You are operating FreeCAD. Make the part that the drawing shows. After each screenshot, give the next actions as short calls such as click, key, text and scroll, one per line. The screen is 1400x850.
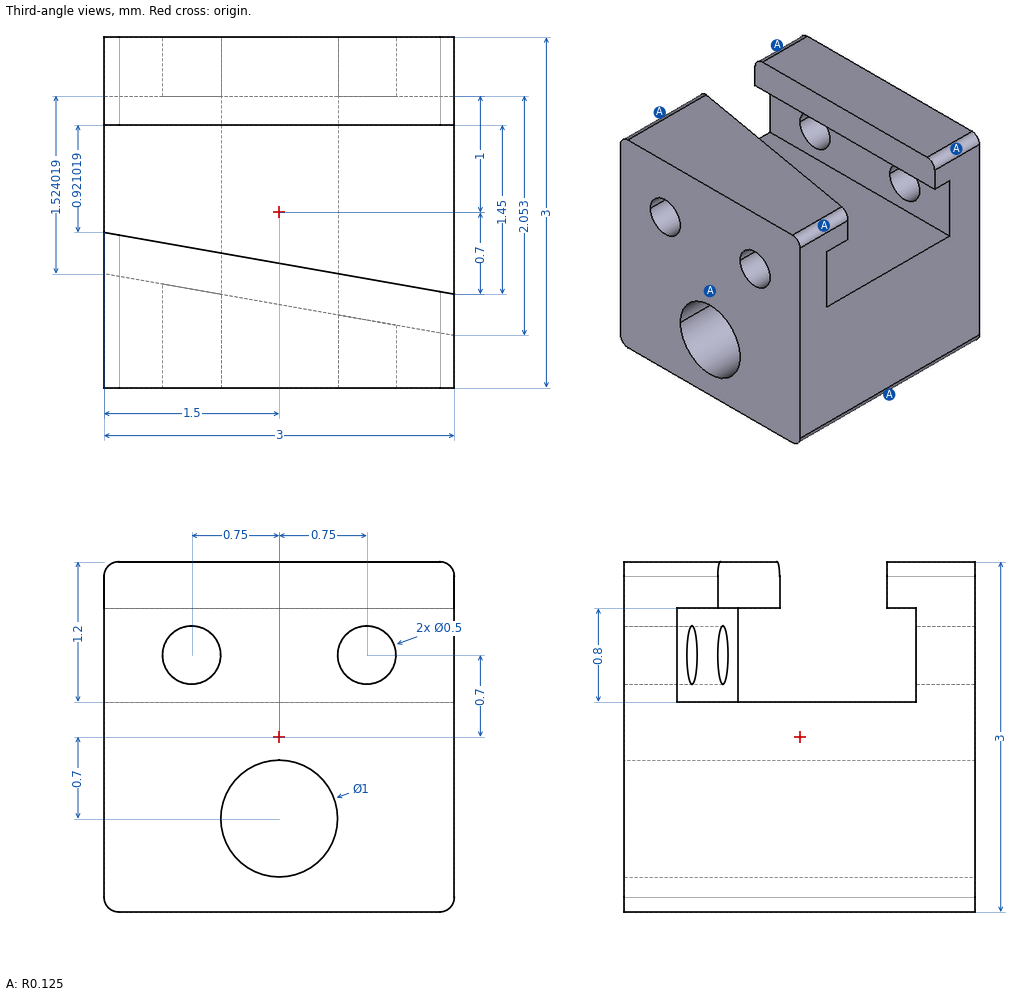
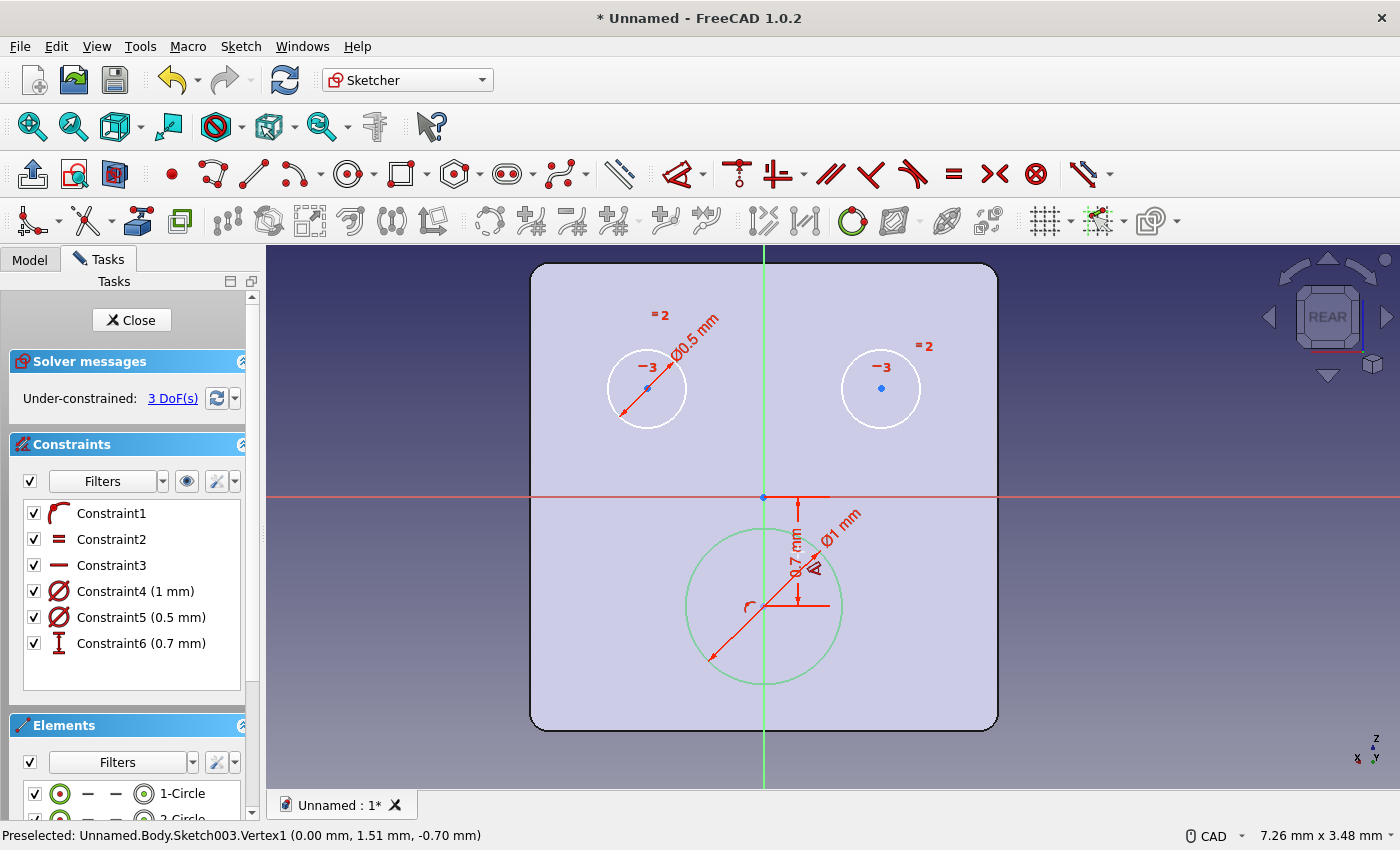
click(647, 389)
click(613, 443)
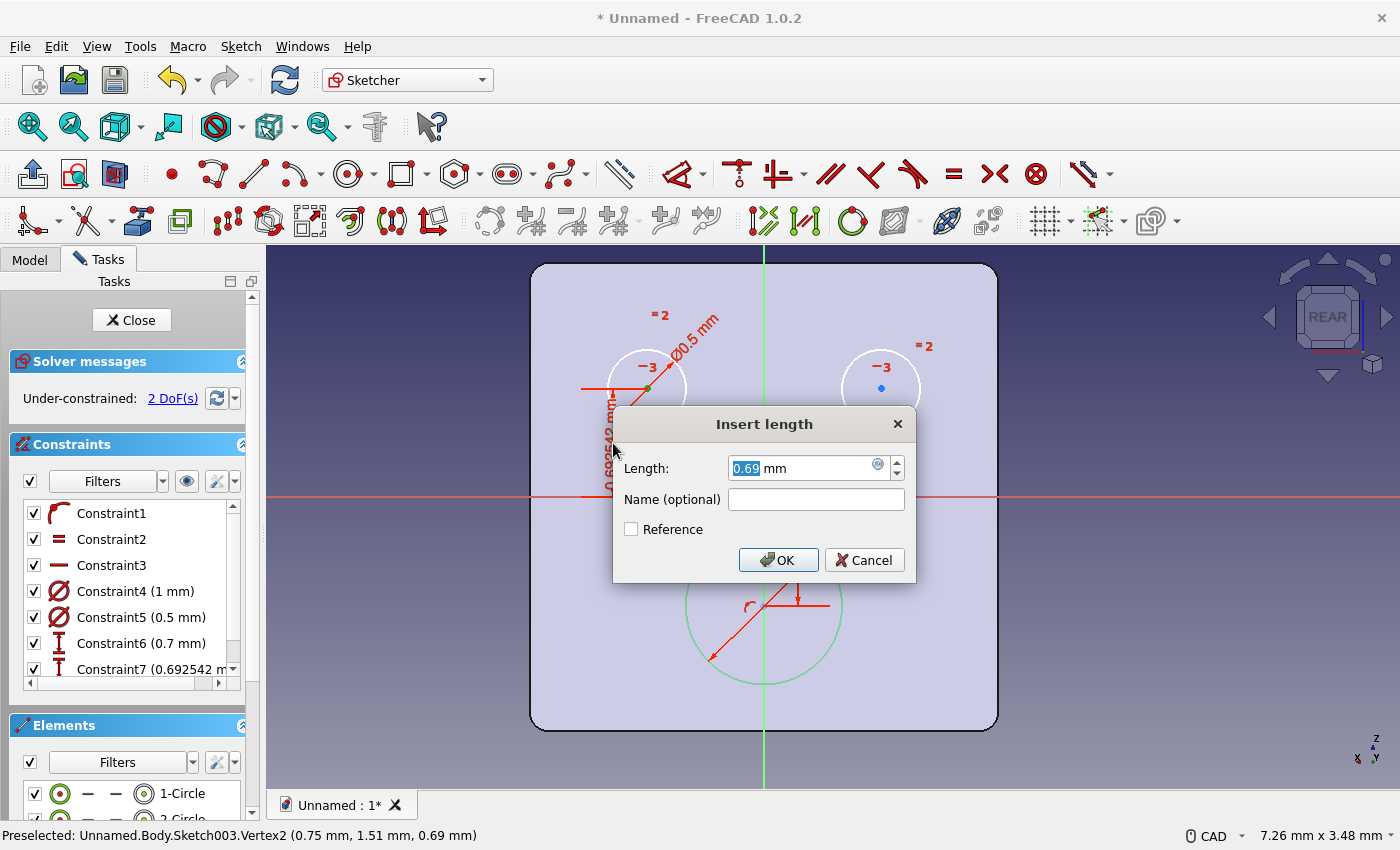
text(0.7)
key(Return)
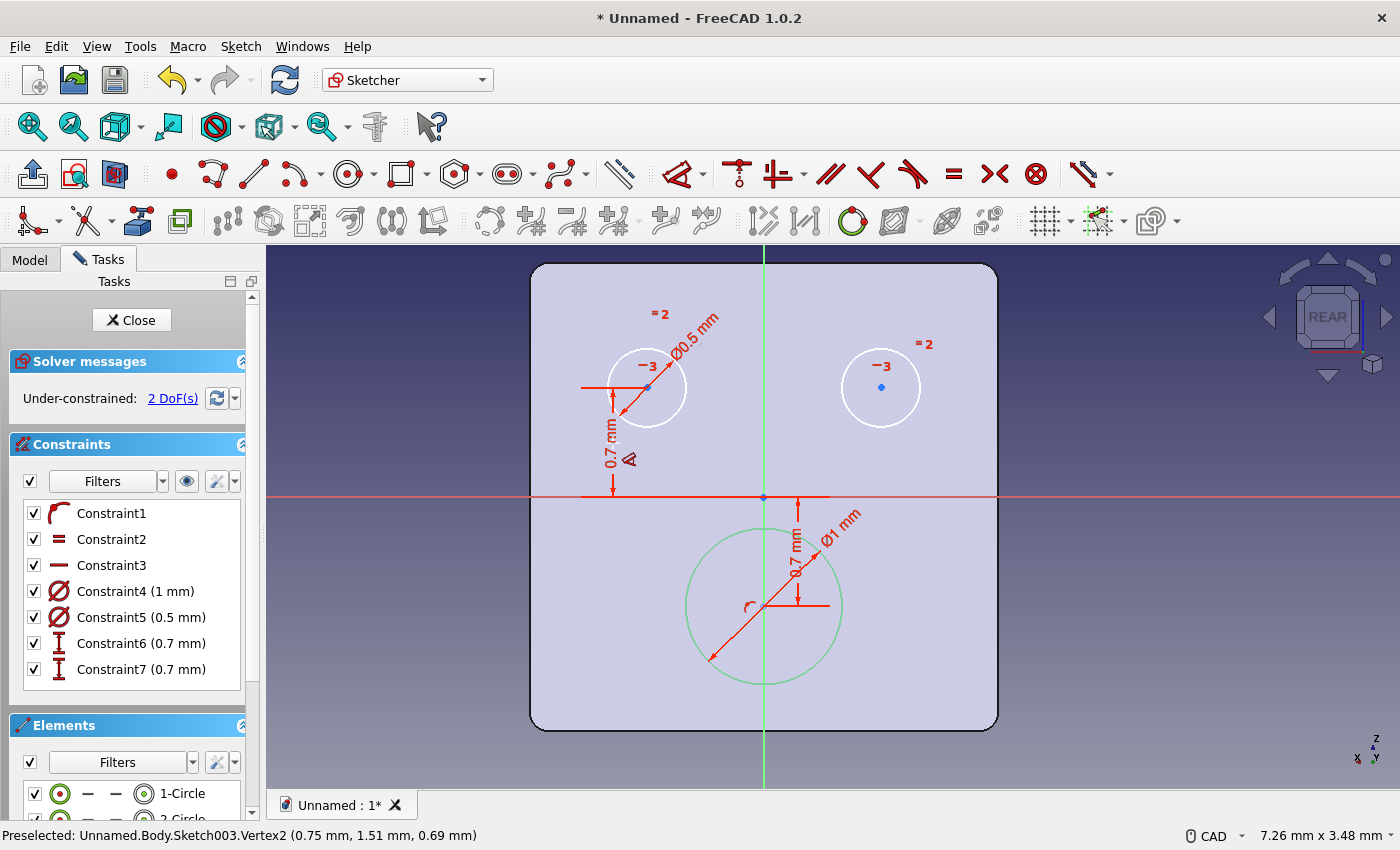
click(647, 388)
click(705, 531)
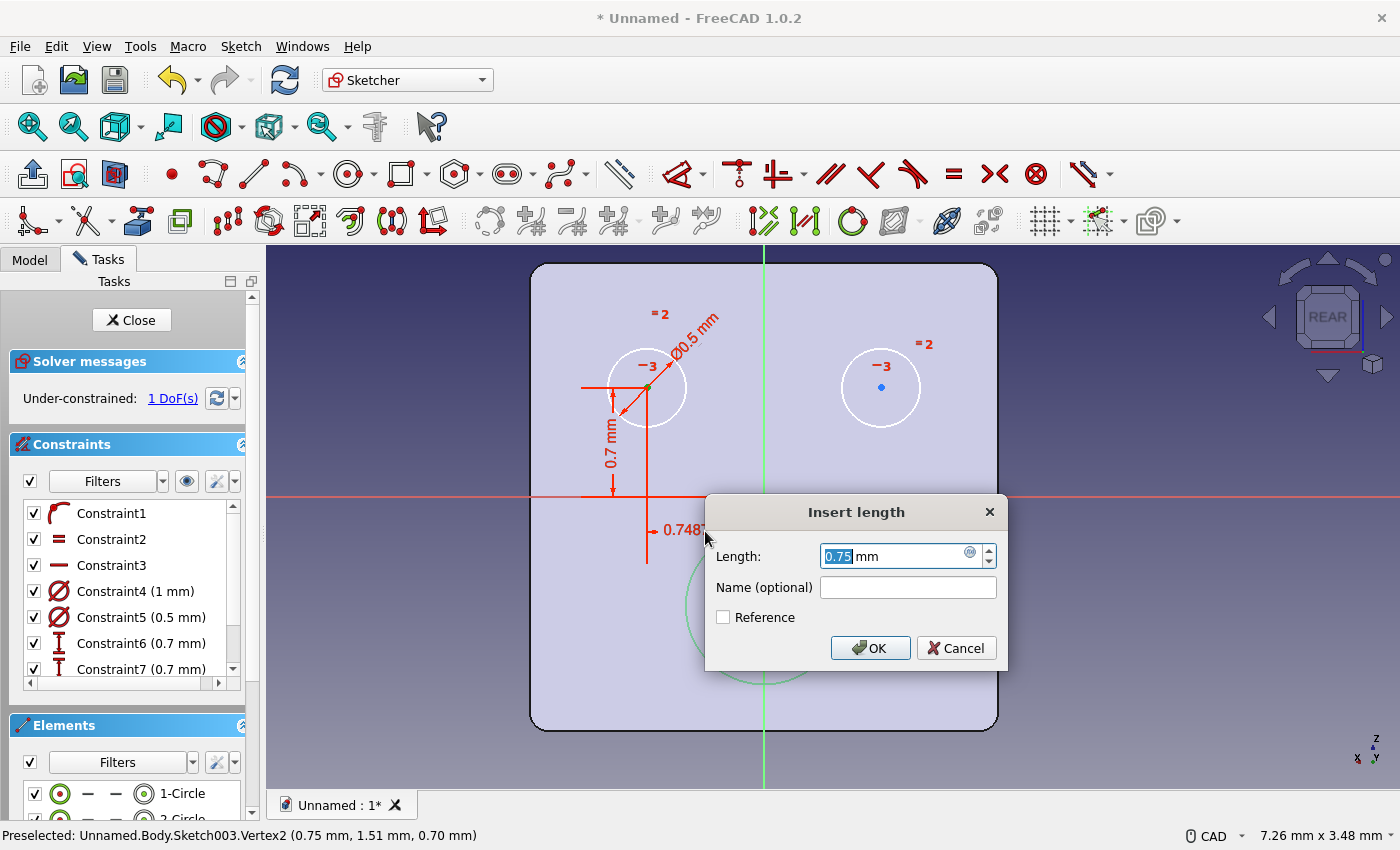
text(0.75)
key(Return)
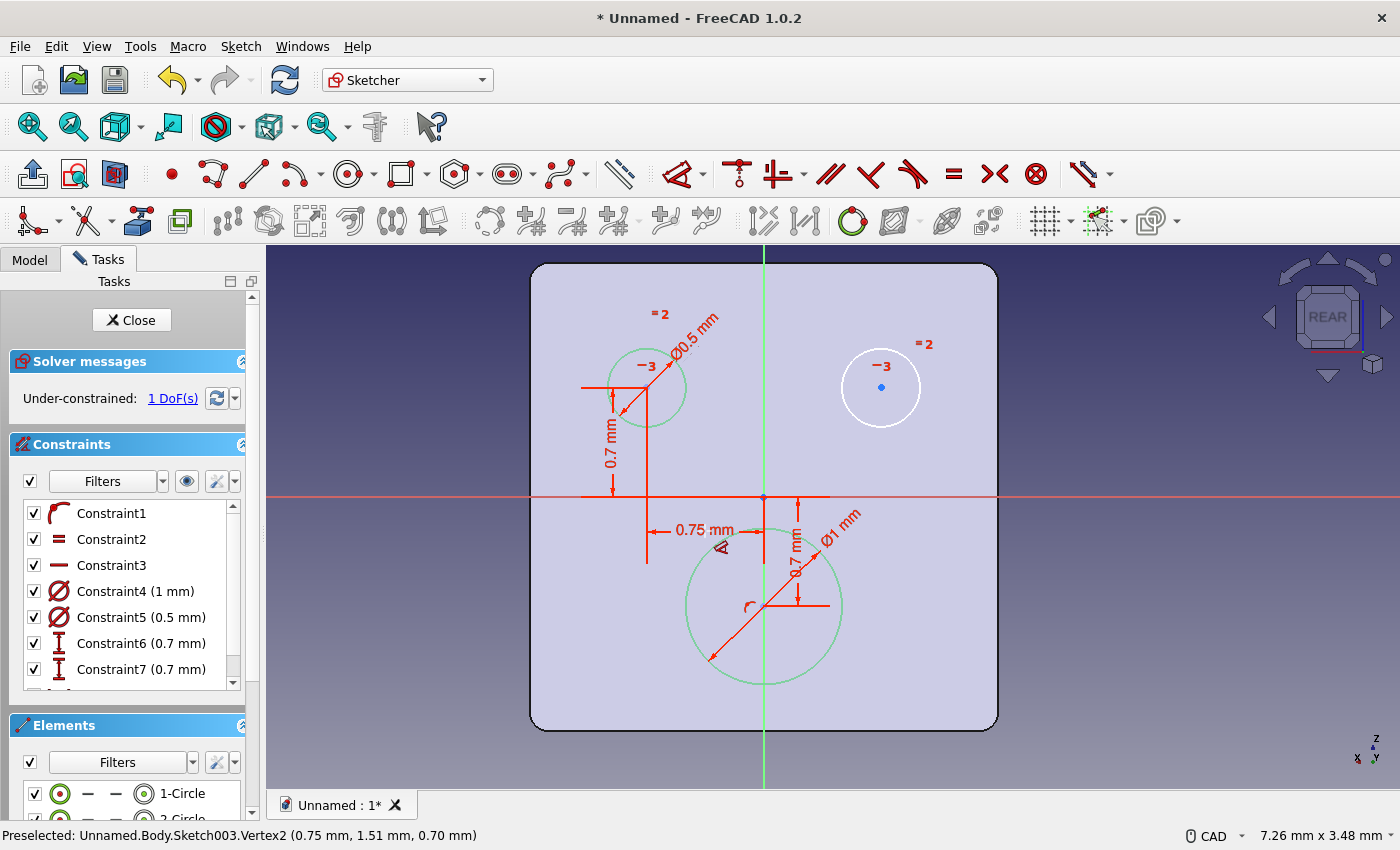
click(881, 388)
click(822, 354)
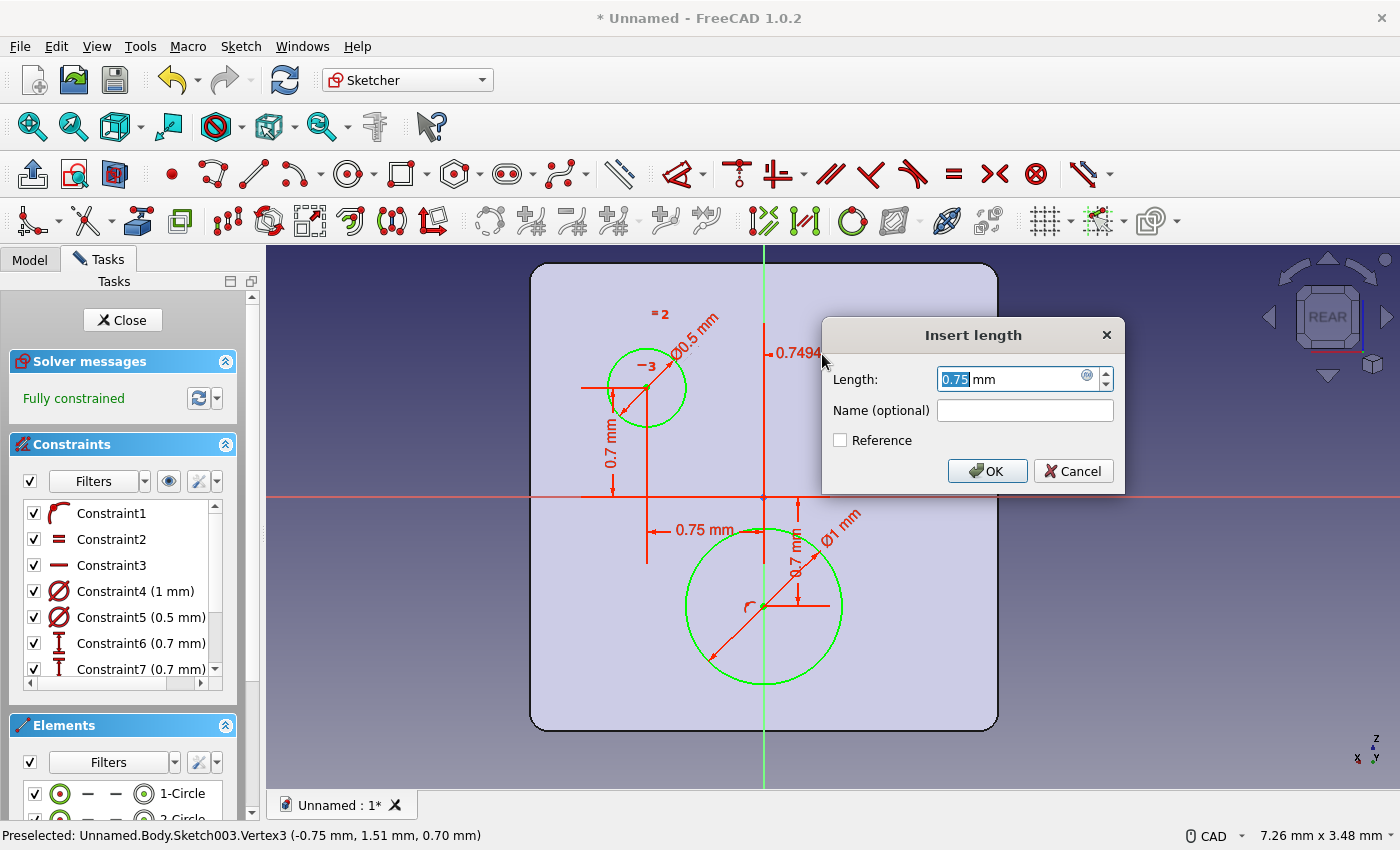
text(0.75)
key(Return)
key(Escape)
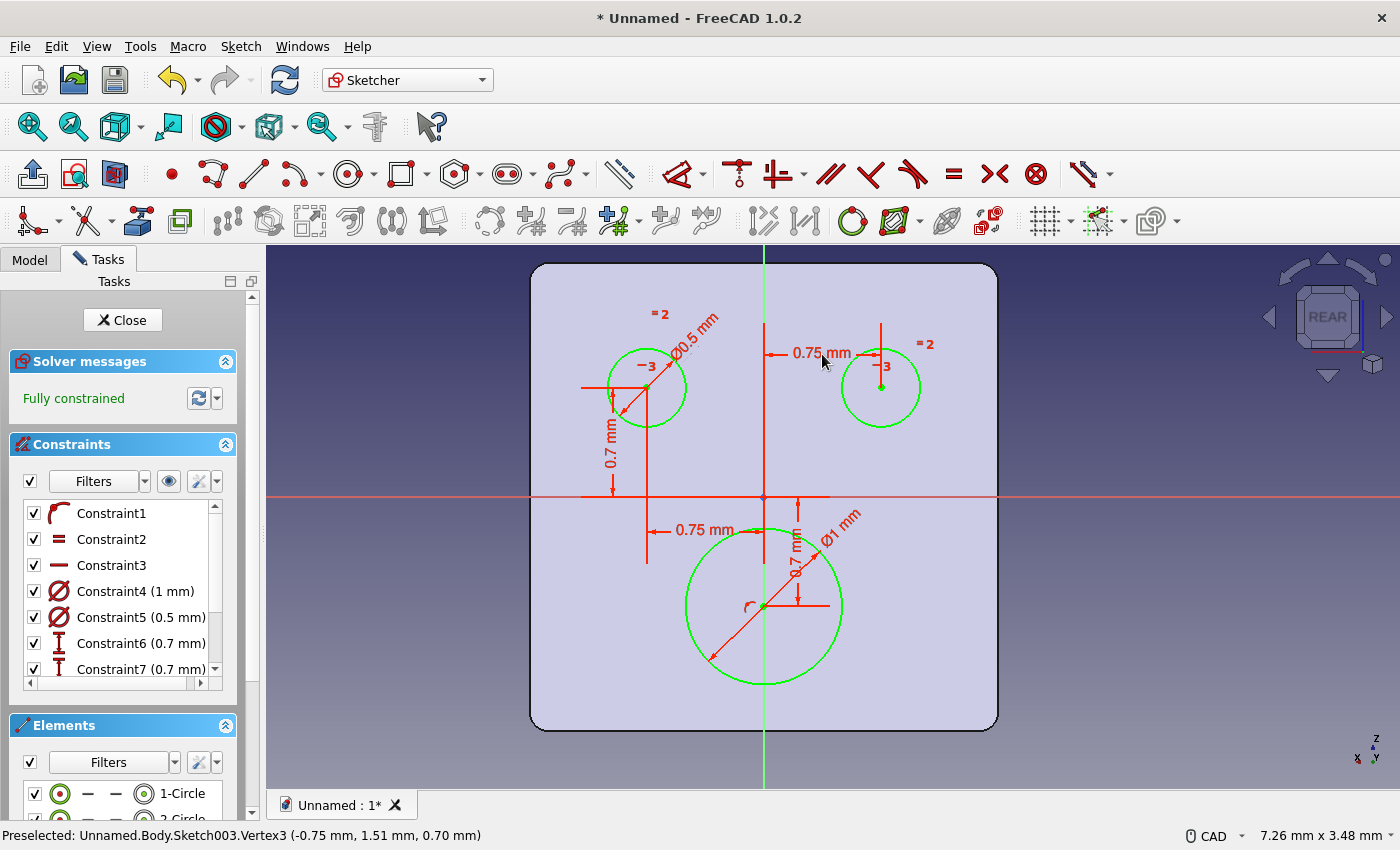
click(123, 320)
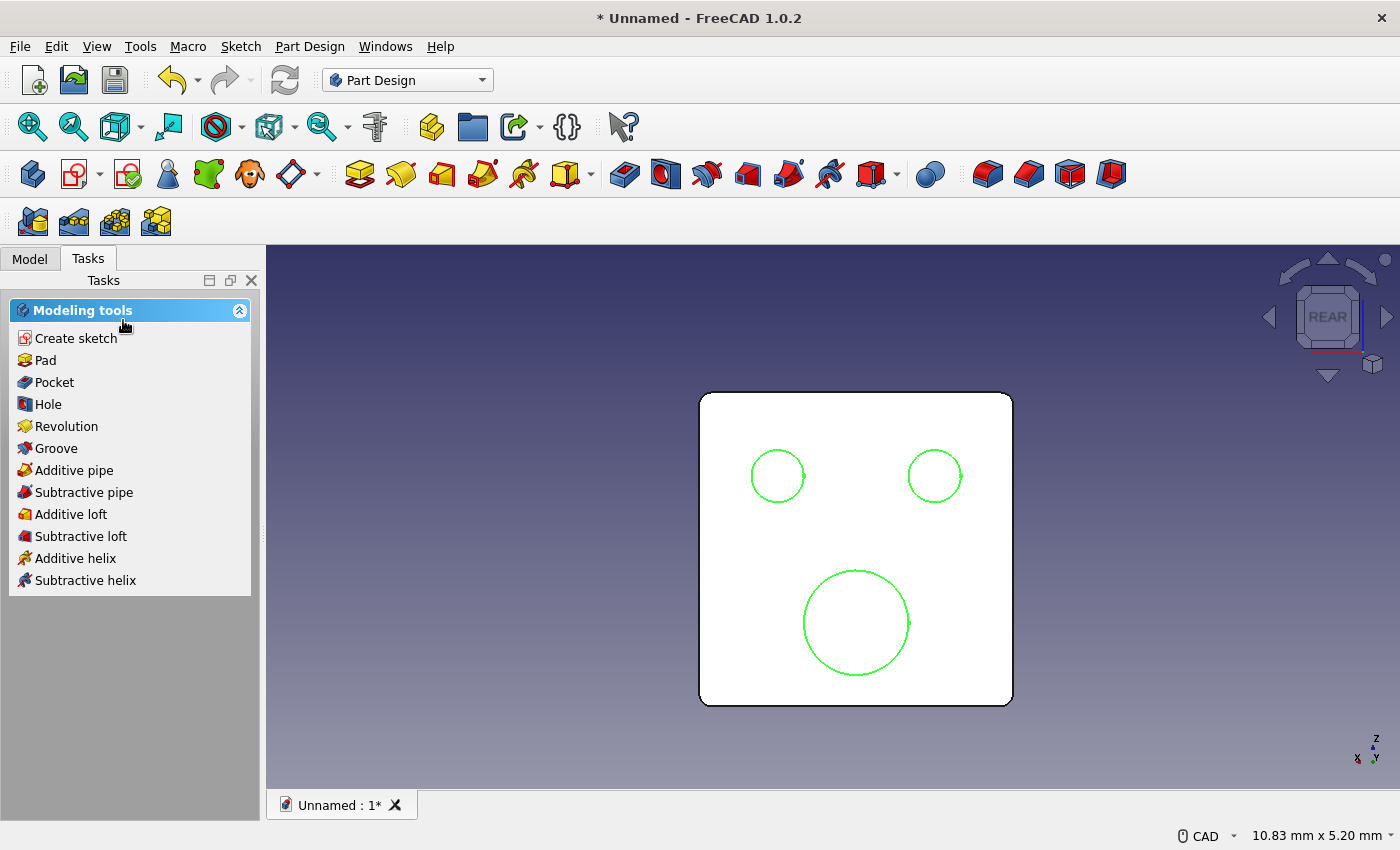
click(625, 174)